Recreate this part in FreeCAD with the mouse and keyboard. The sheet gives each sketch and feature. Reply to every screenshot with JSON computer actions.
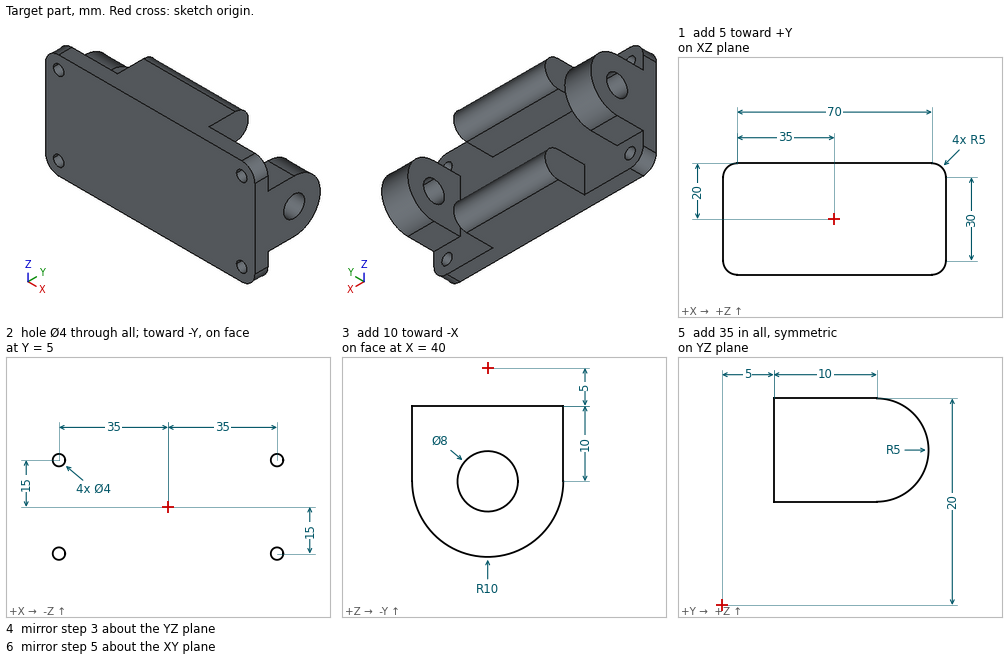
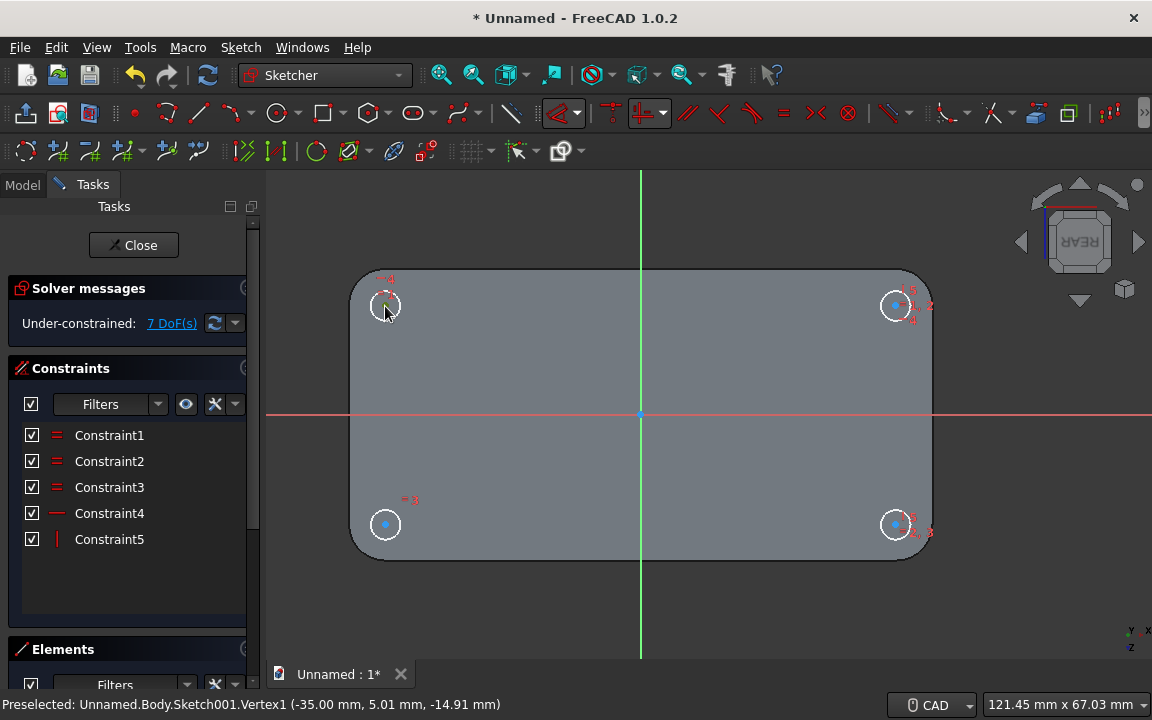
{"action": "left_click", "coordinate": [386, 525]}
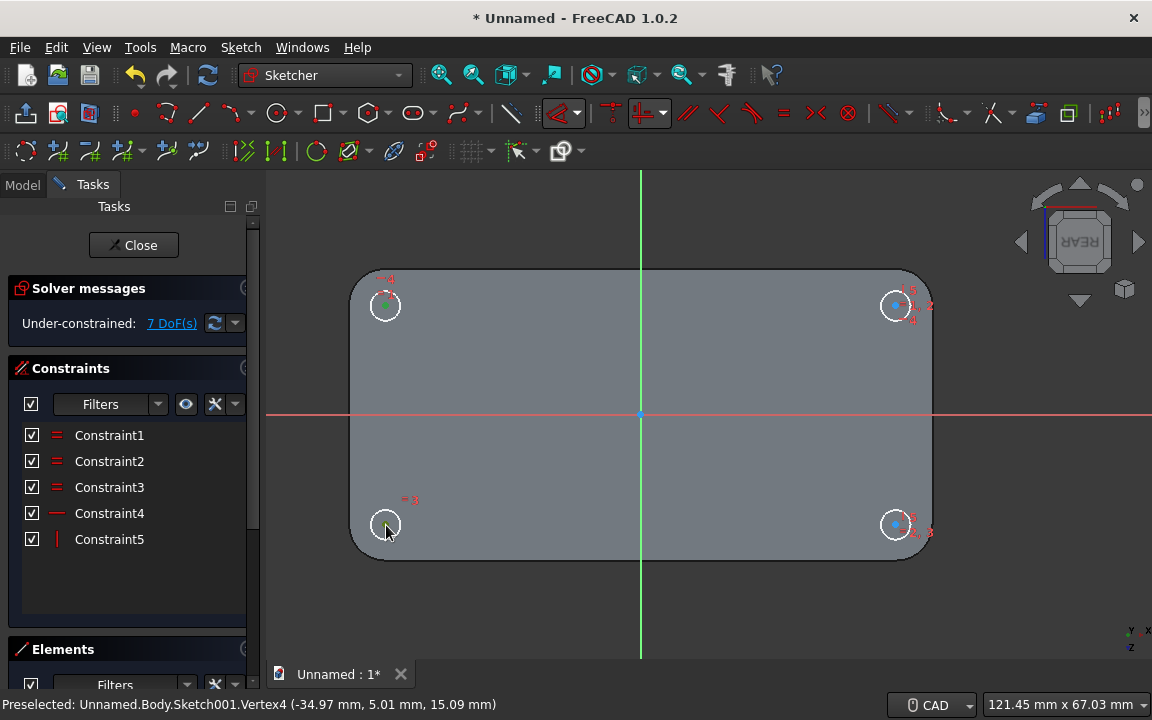
{"action": "key", "text": "v"}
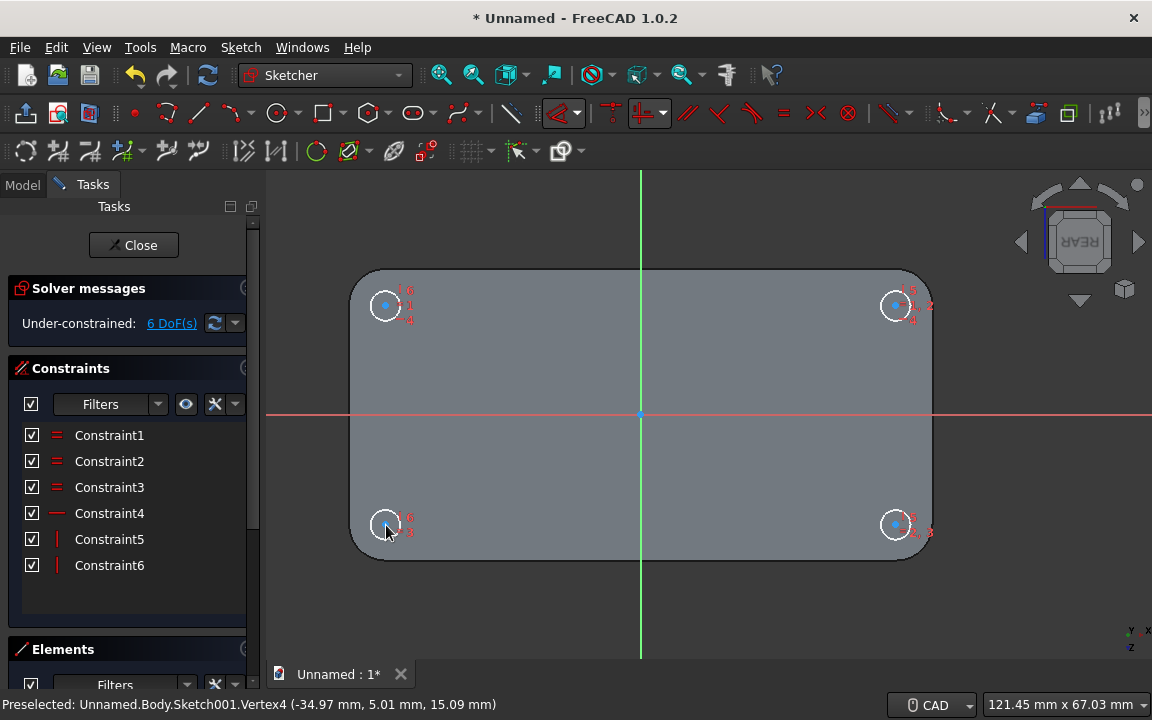
{"action": "left_click", "coordinate": [896, 525]}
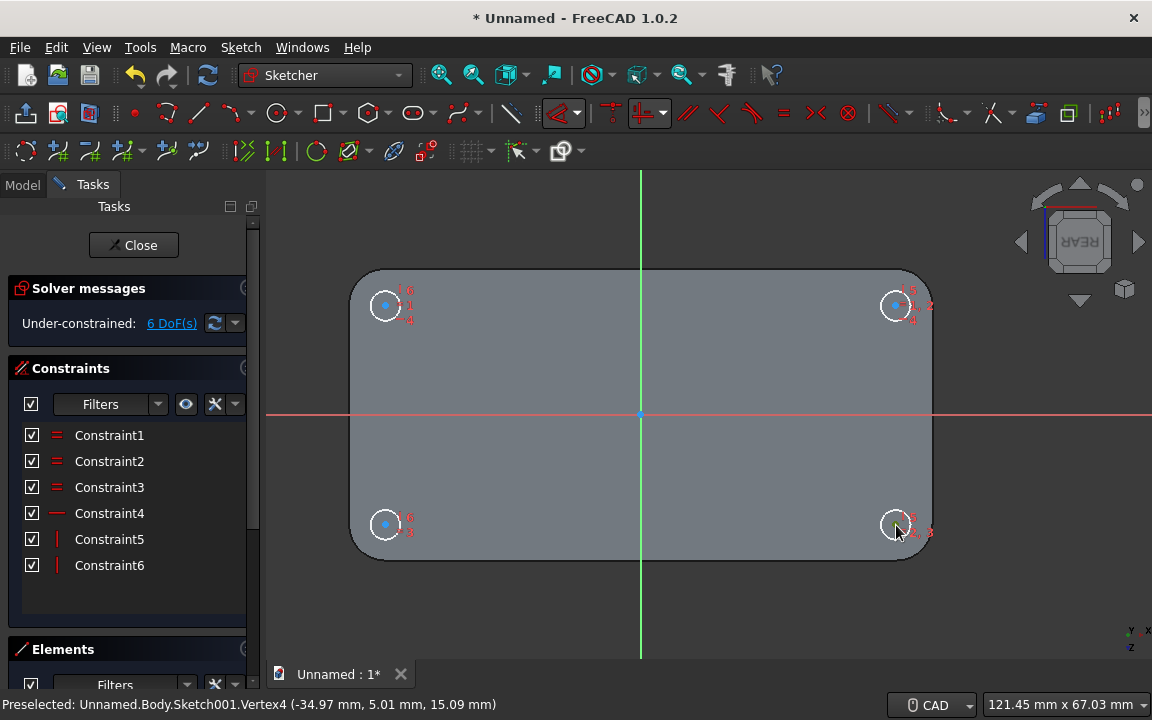
{"action": "left_click", "coordinate": [385, 525]}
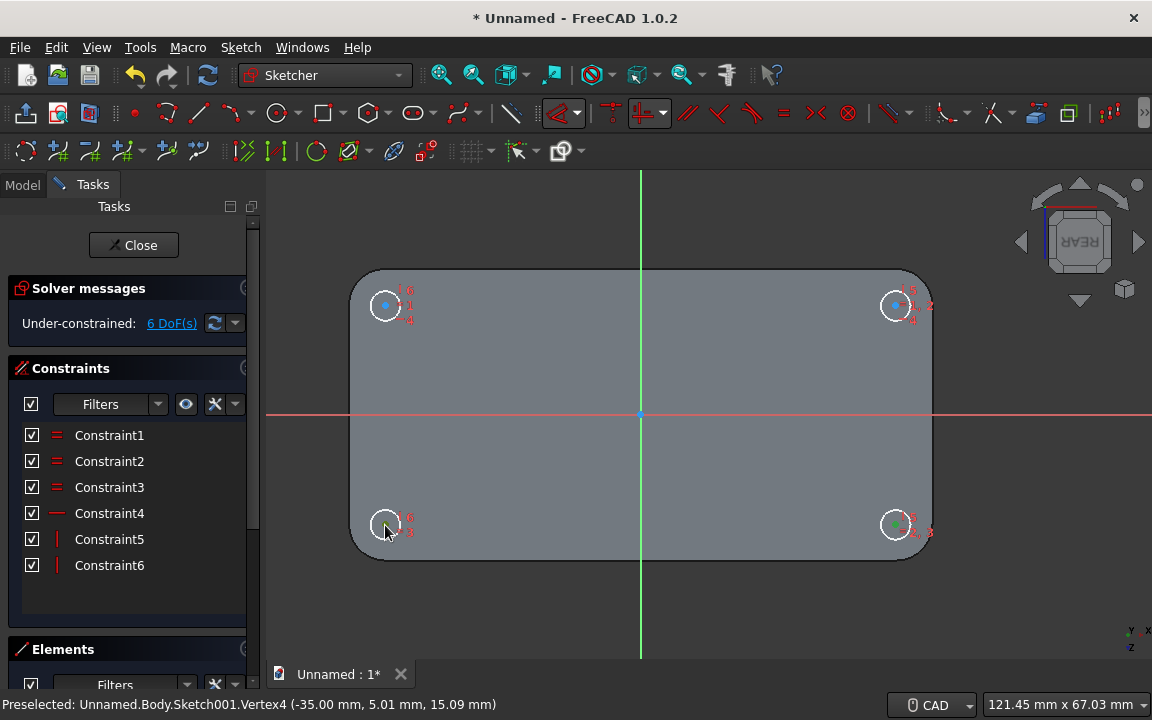
{"action": "left_click", "coordinate": [666, 114]}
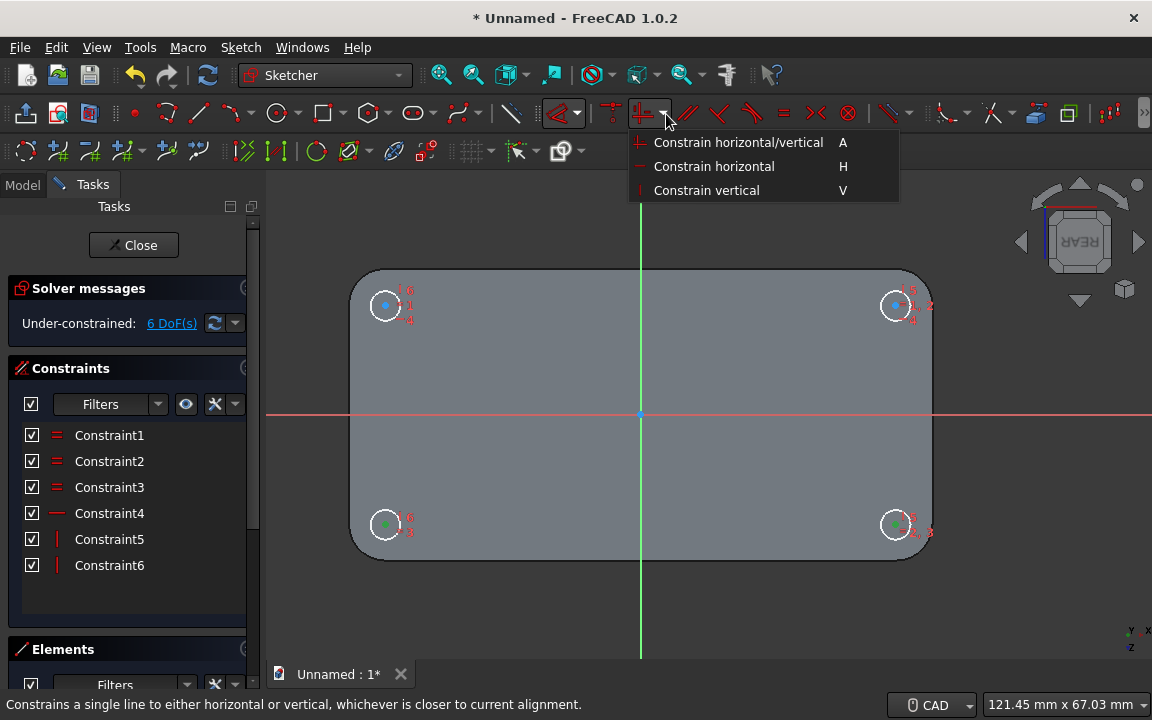
{"action": "left_click", "coordinate": [764, 166]}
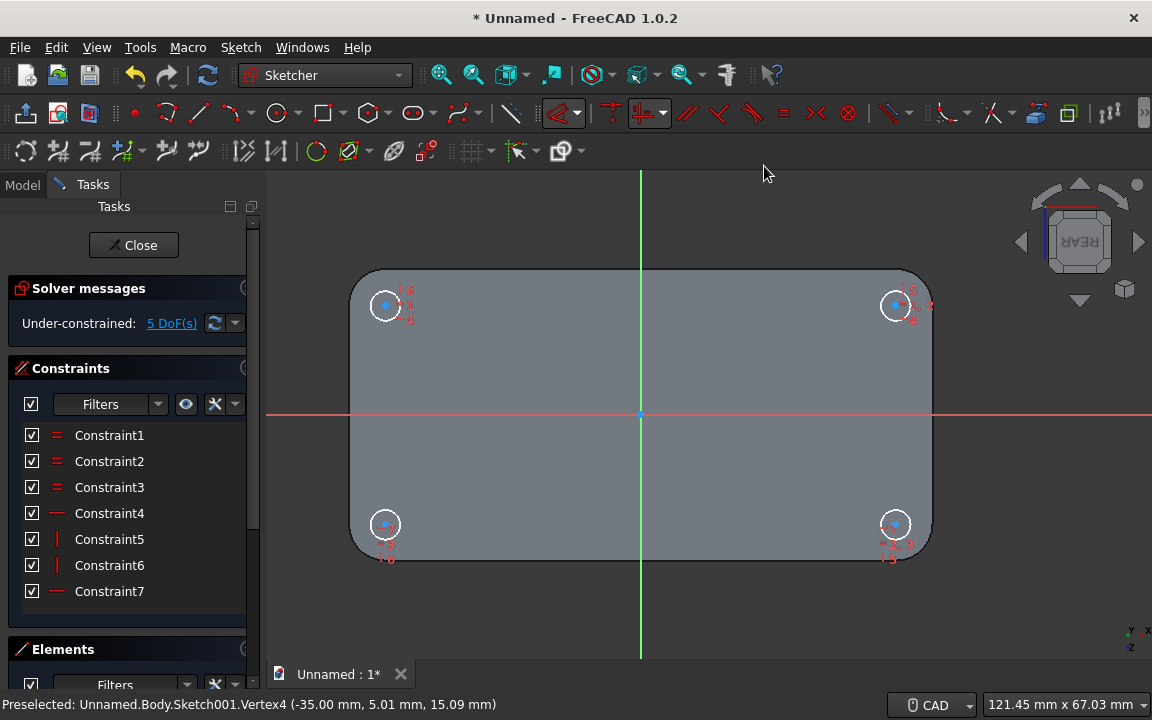
{"action": "scroll", "coordinate": [396, 296], "scroll_direction": "up", "scroll_amount": 2}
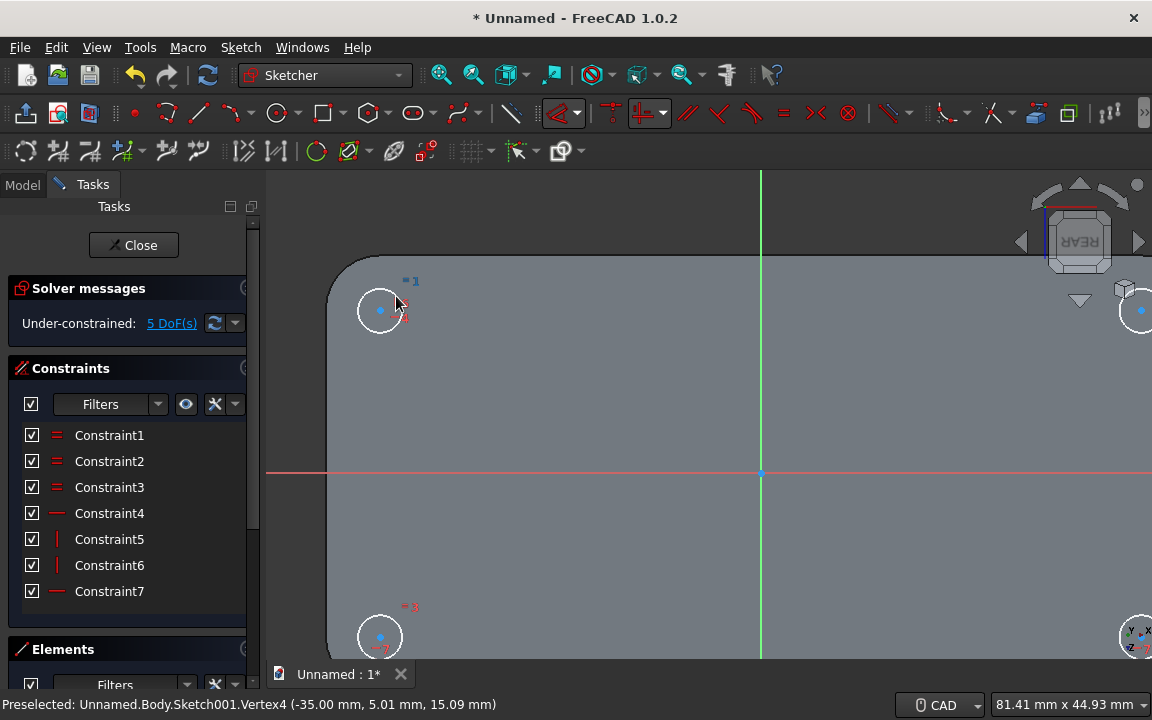
{"action": "left_click", "coordinate": [364, 295]}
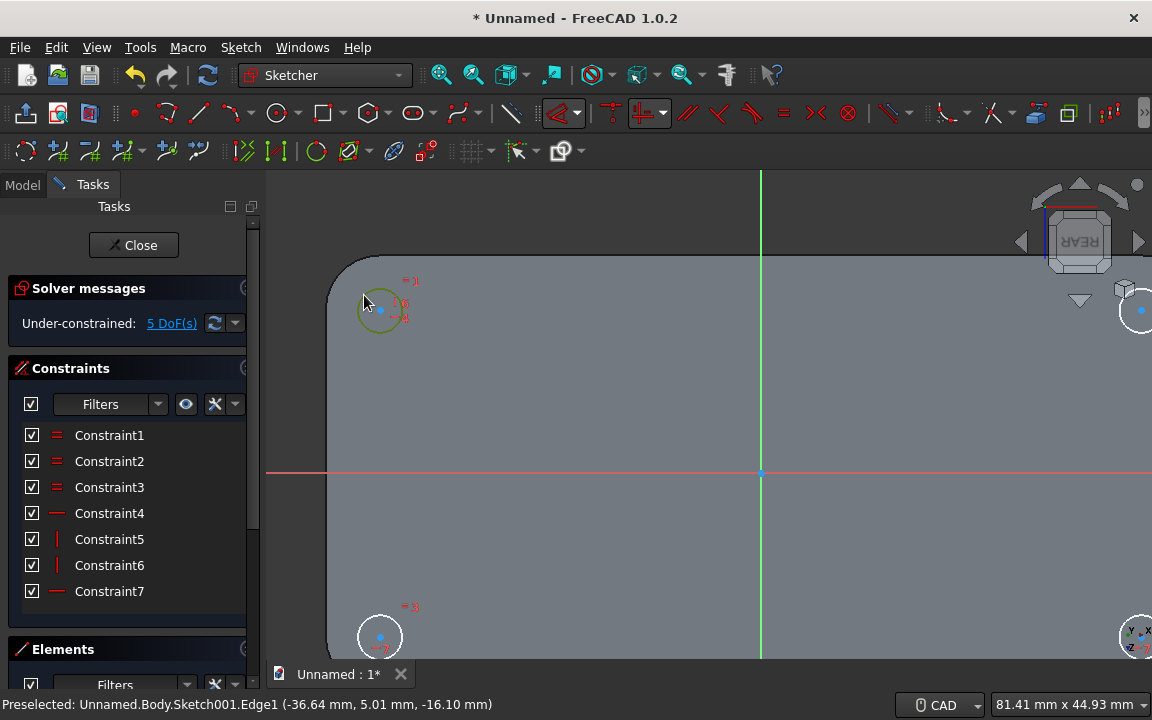
{"action": "key", "text": "k o"}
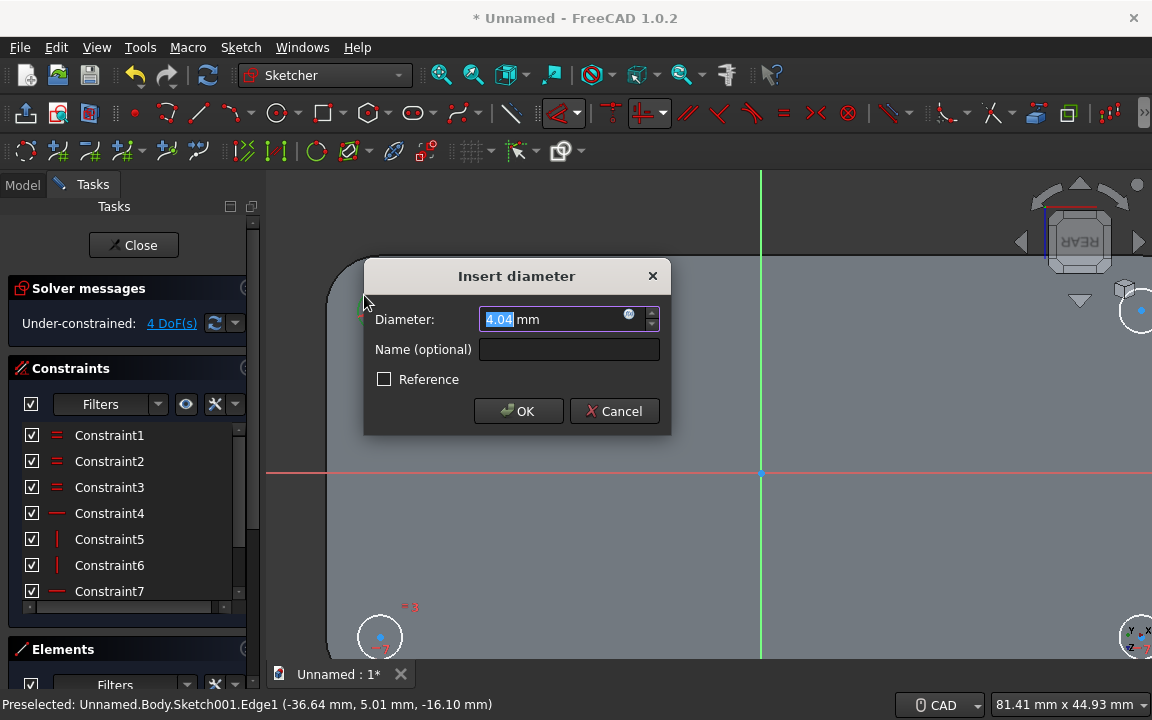
{"action": "type", "text": "4"}
{"action": "key", "text": "Return"}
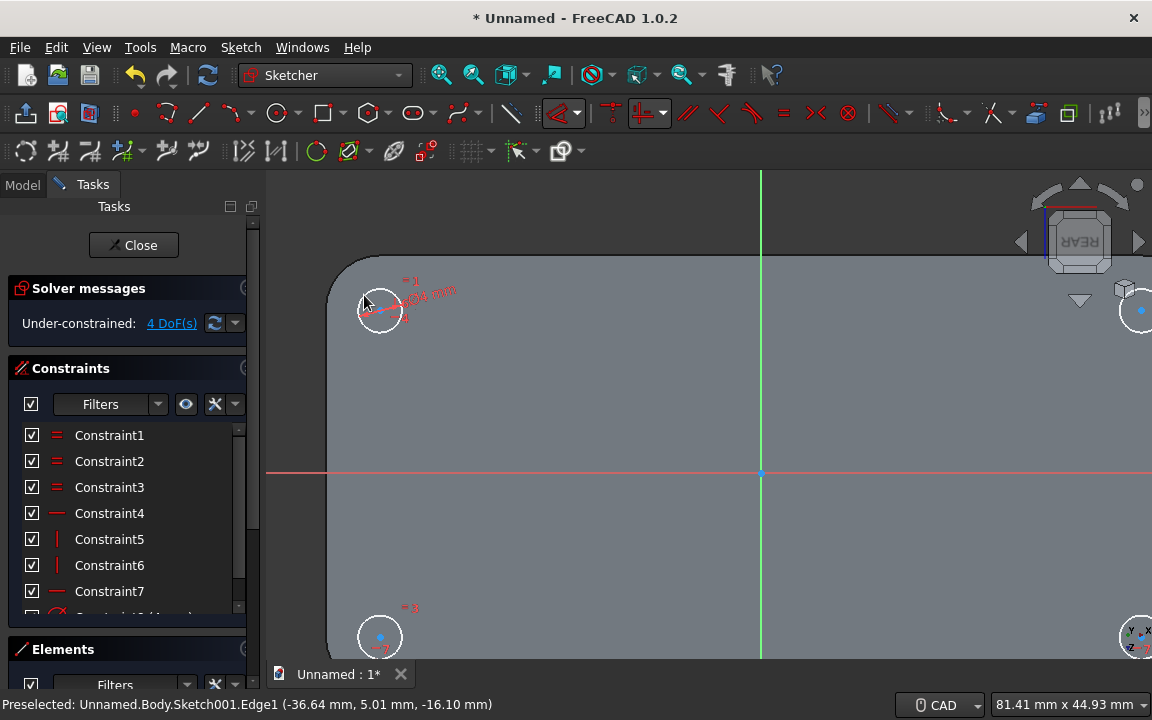
{"action": "left_click", "coordinate": [380, 311]}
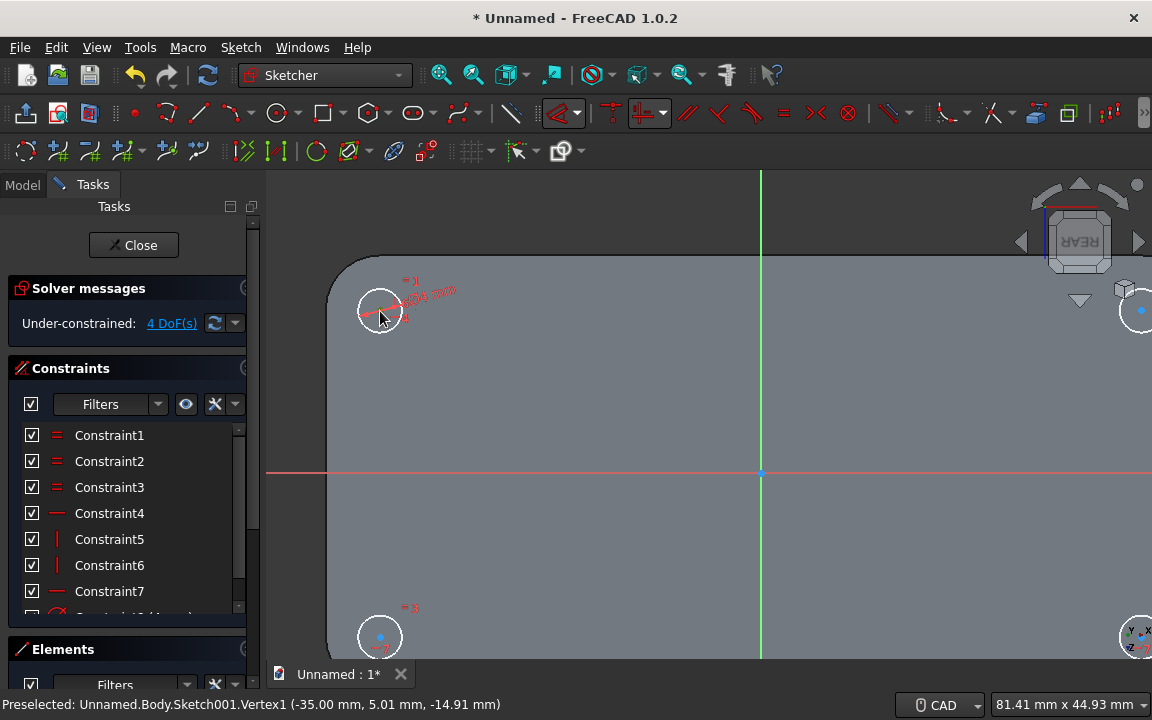
{"action": "key", "text": "l"}